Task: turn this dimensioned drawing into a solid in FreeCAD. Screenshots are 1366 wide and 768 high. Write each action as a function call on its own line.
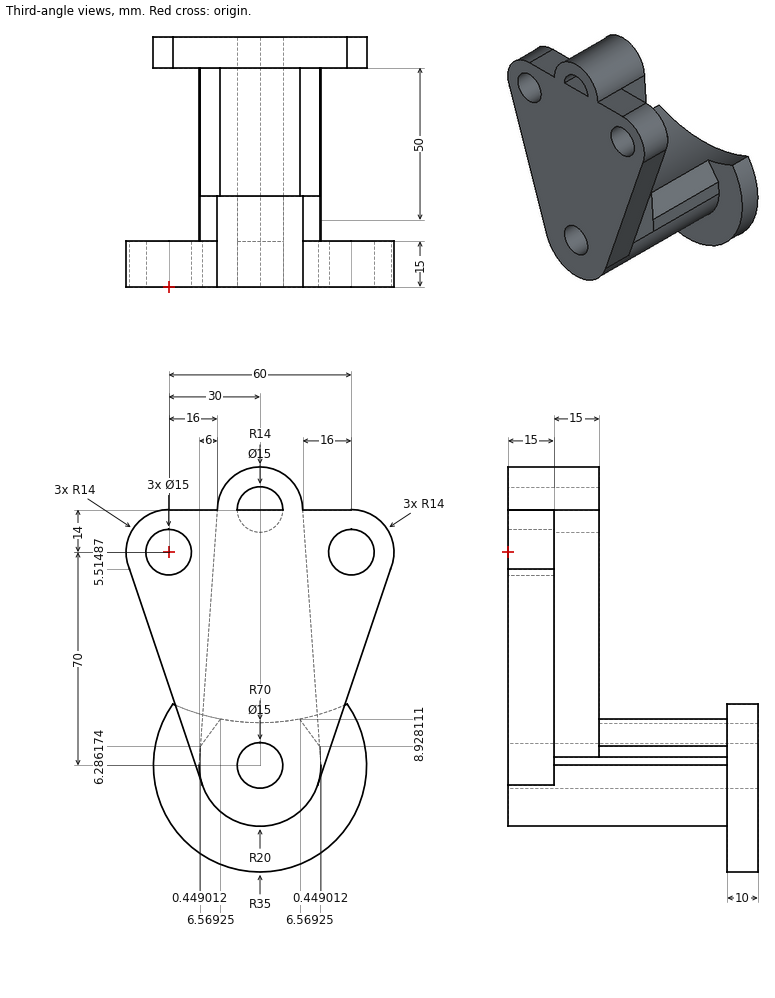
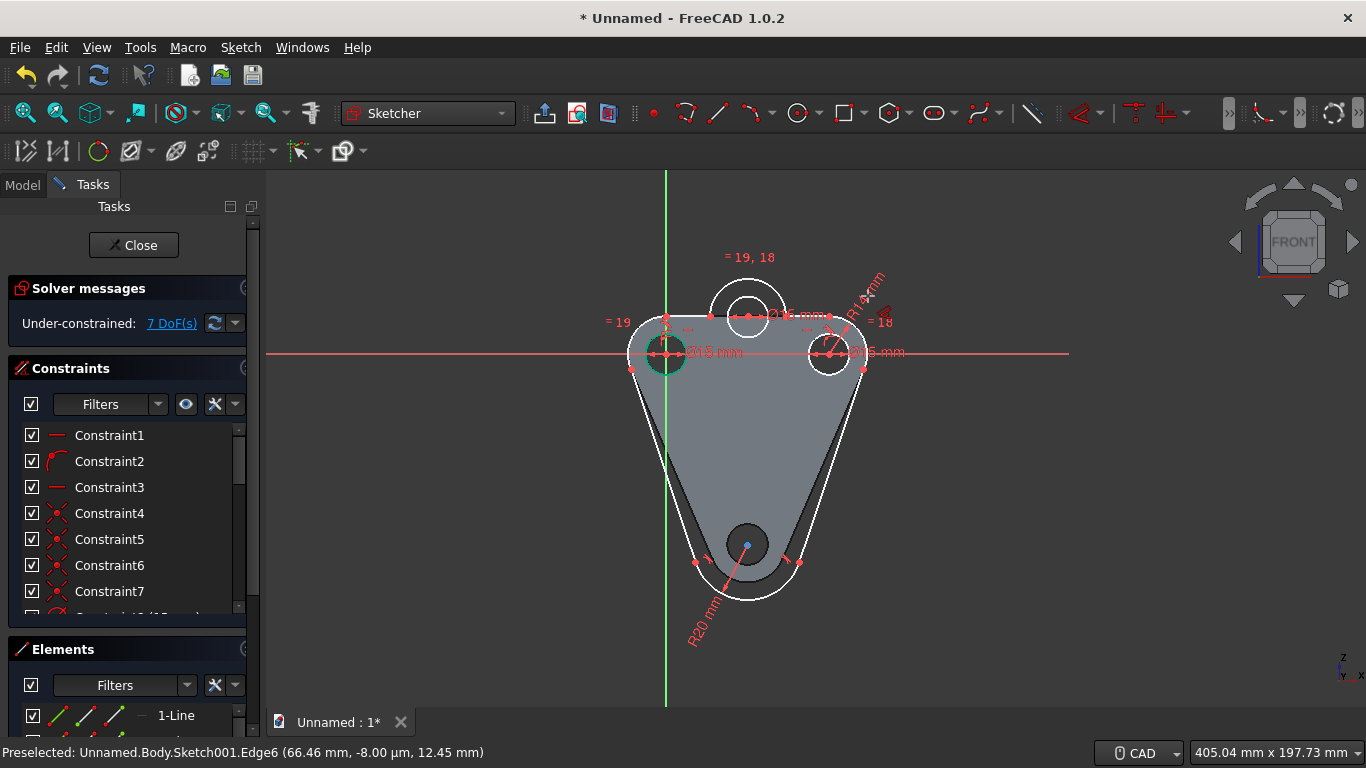
click(816, 316)
click(798, 282)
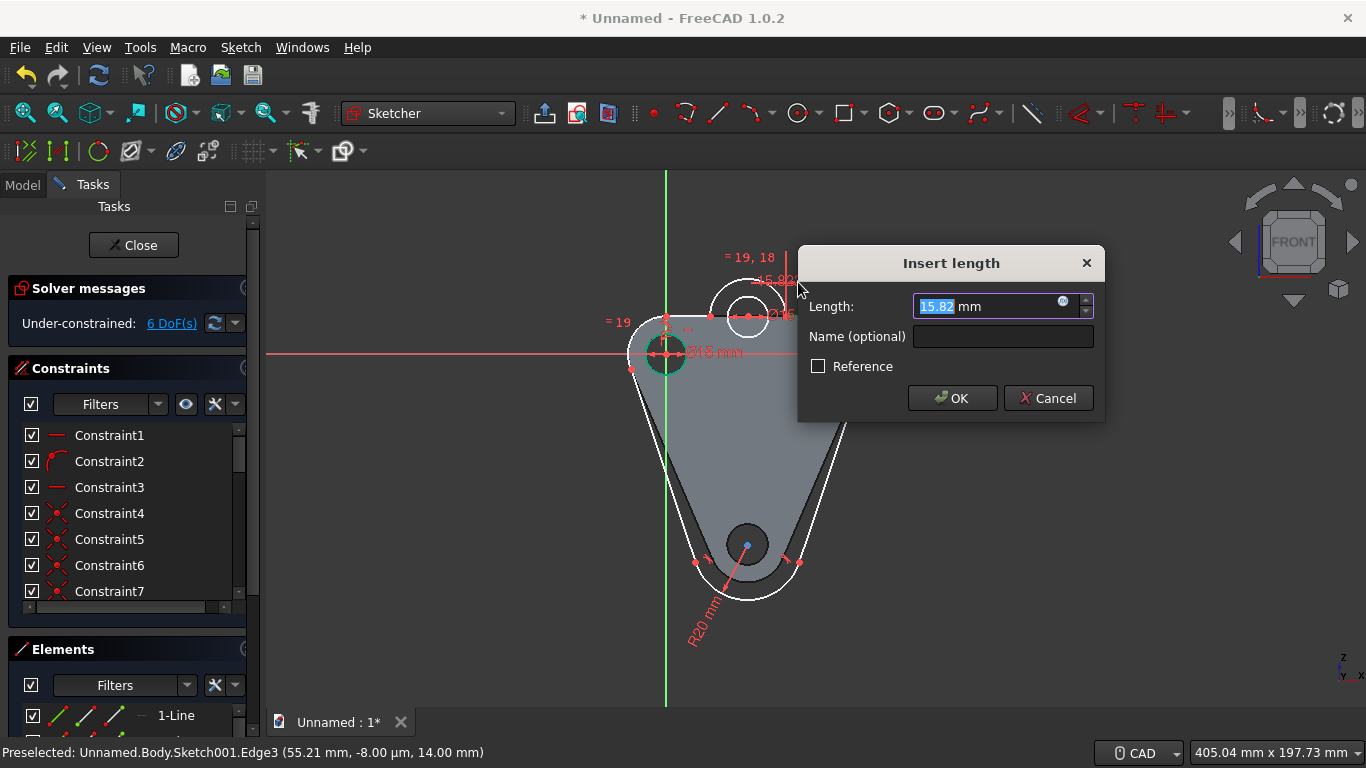
text(16)
key(Return)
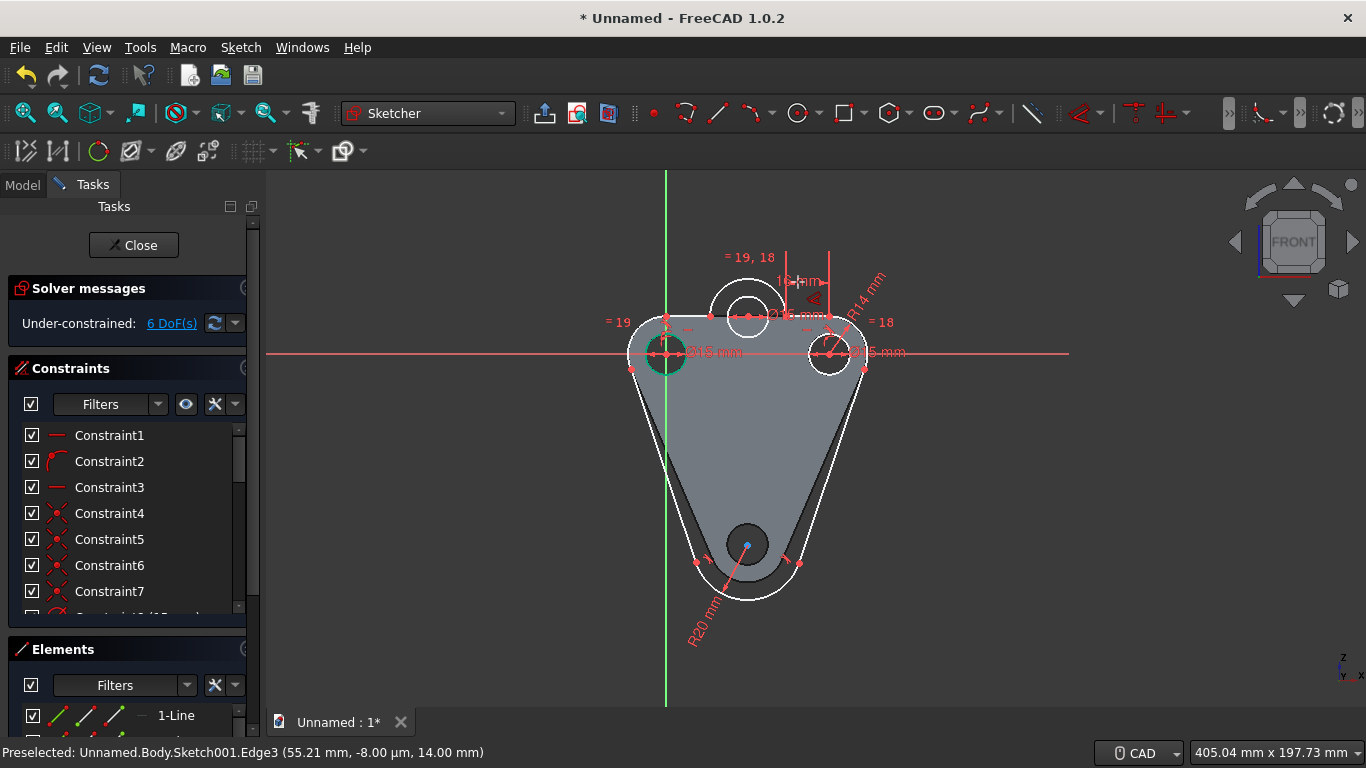
click(697, 316)
click(688, 282)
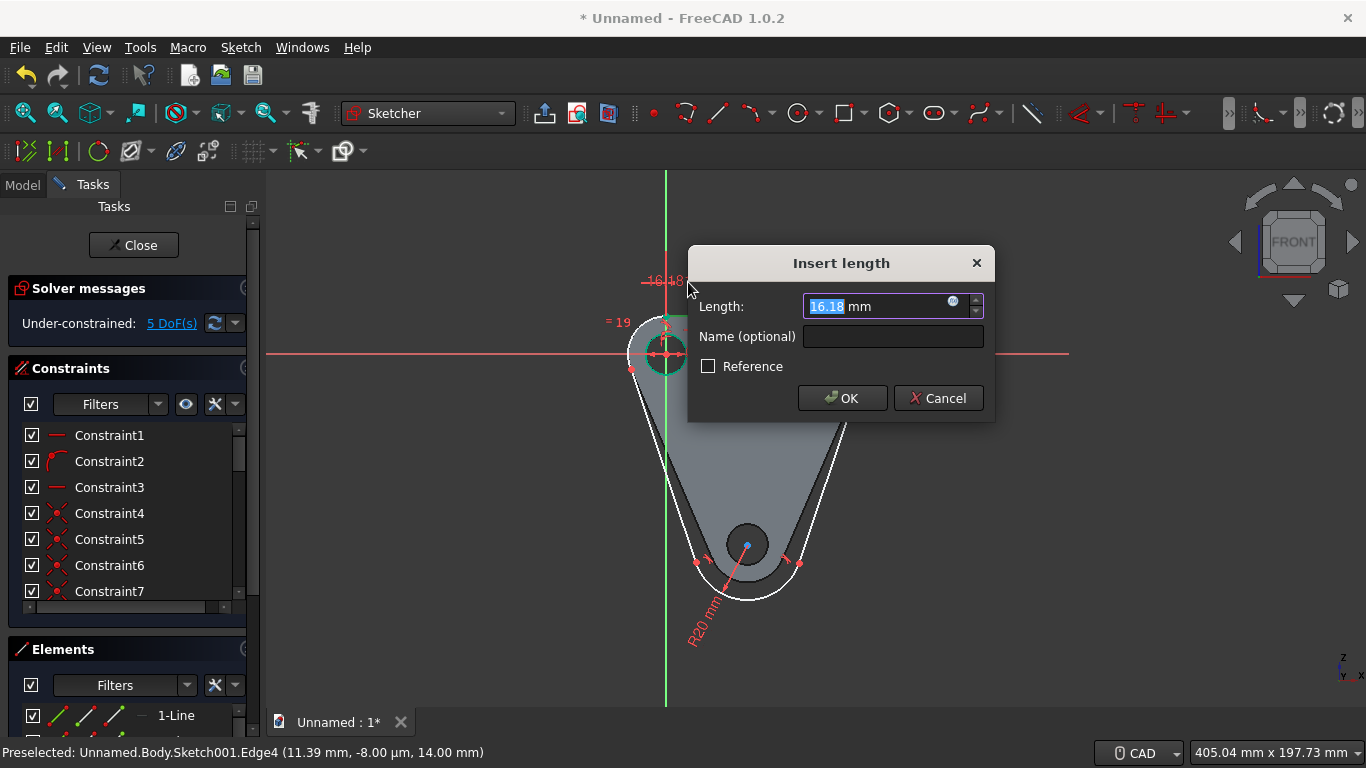
text(16)
key(Return)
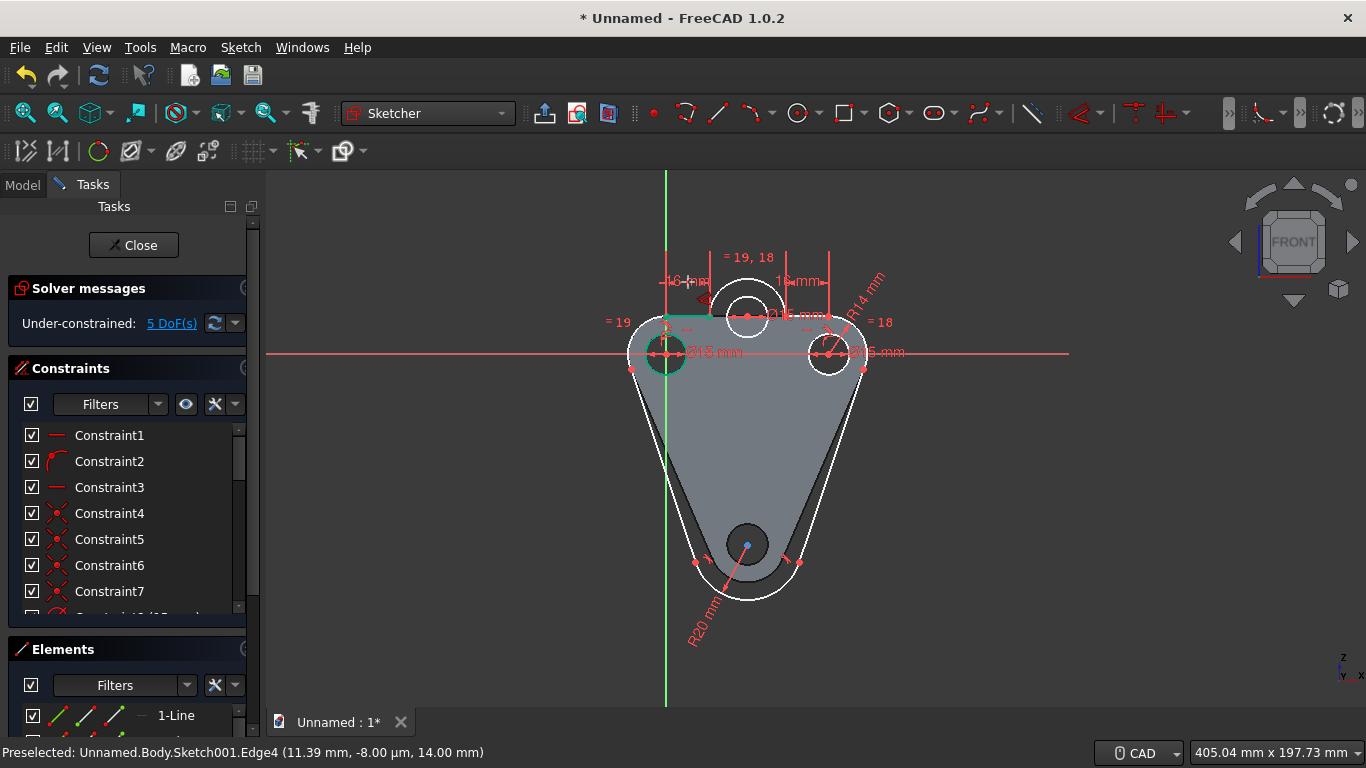
click(748, 317)
click(782, 336)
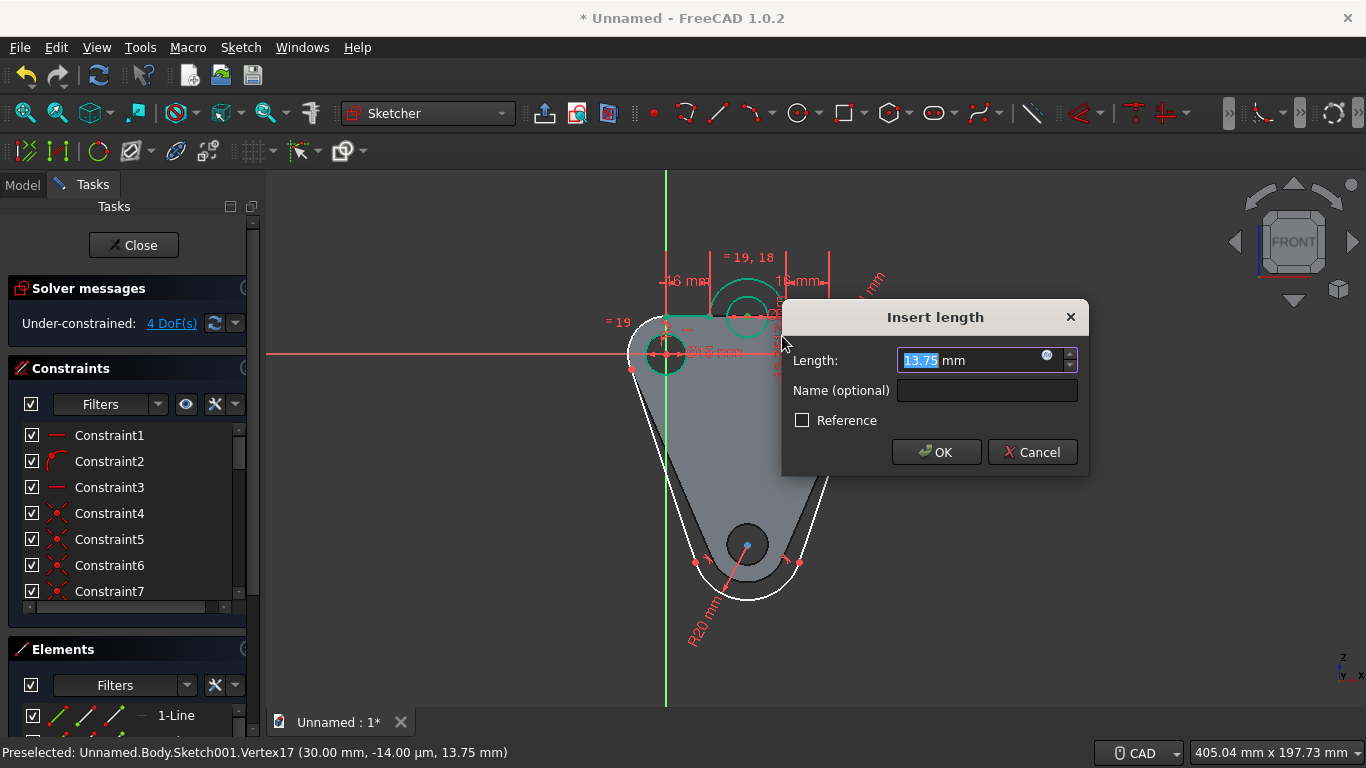
text(14)
key(Return)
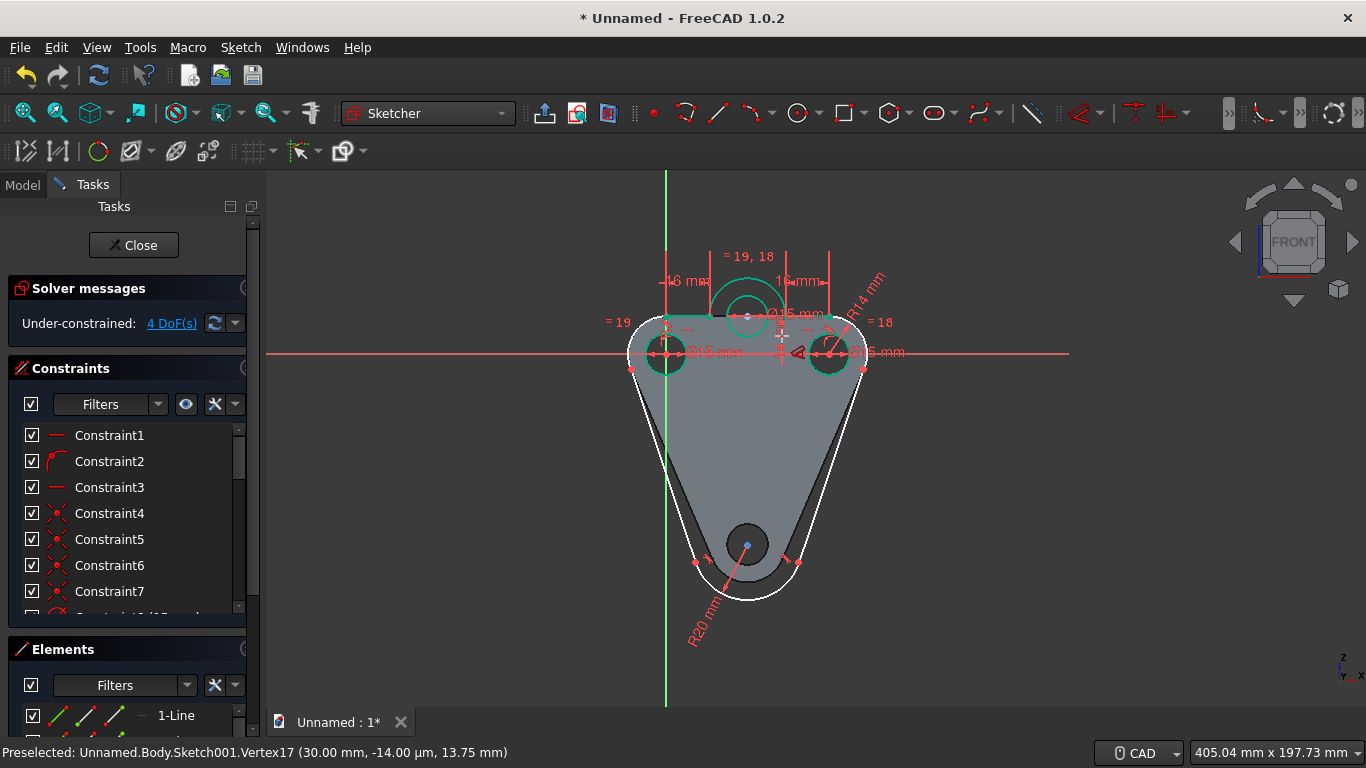
click(747, 546)
click(688, 580)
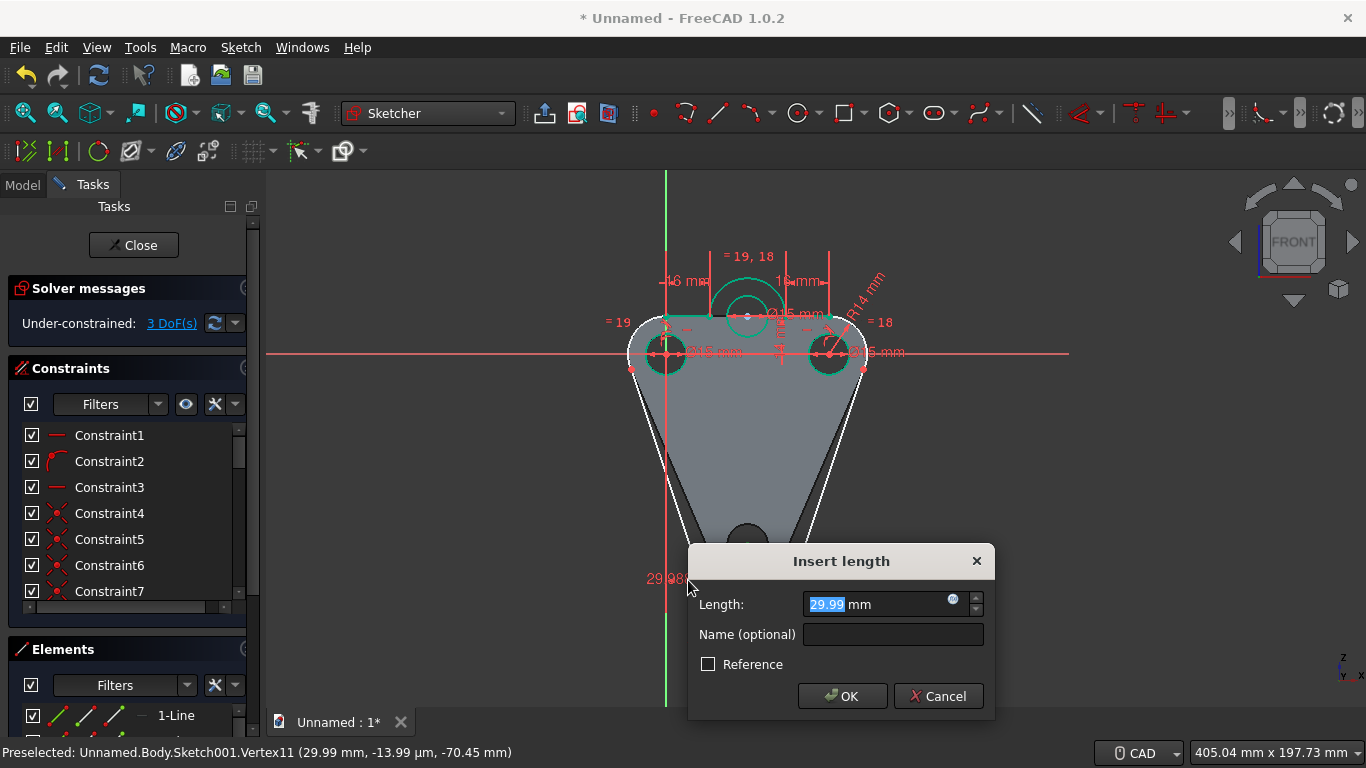
text(30)
key(Return)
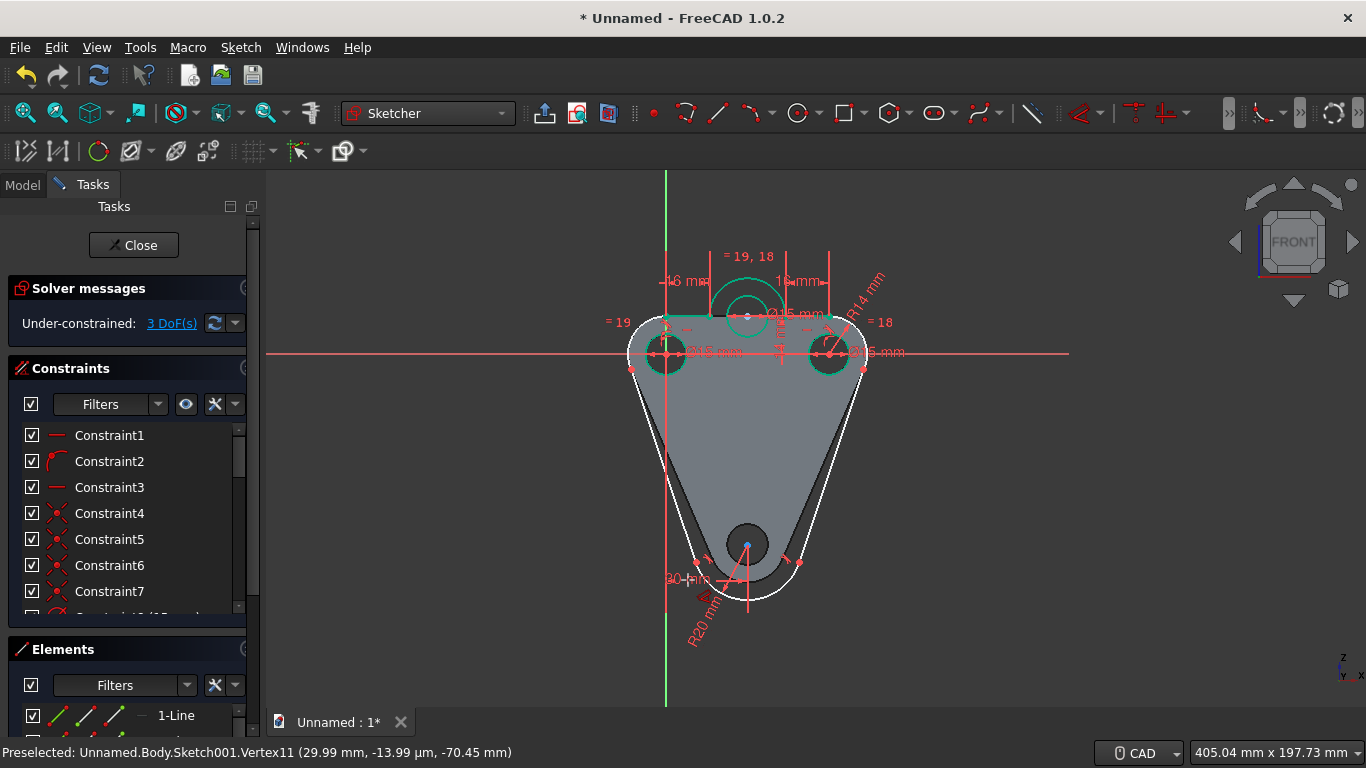
click(748, 546)
click(632, 450)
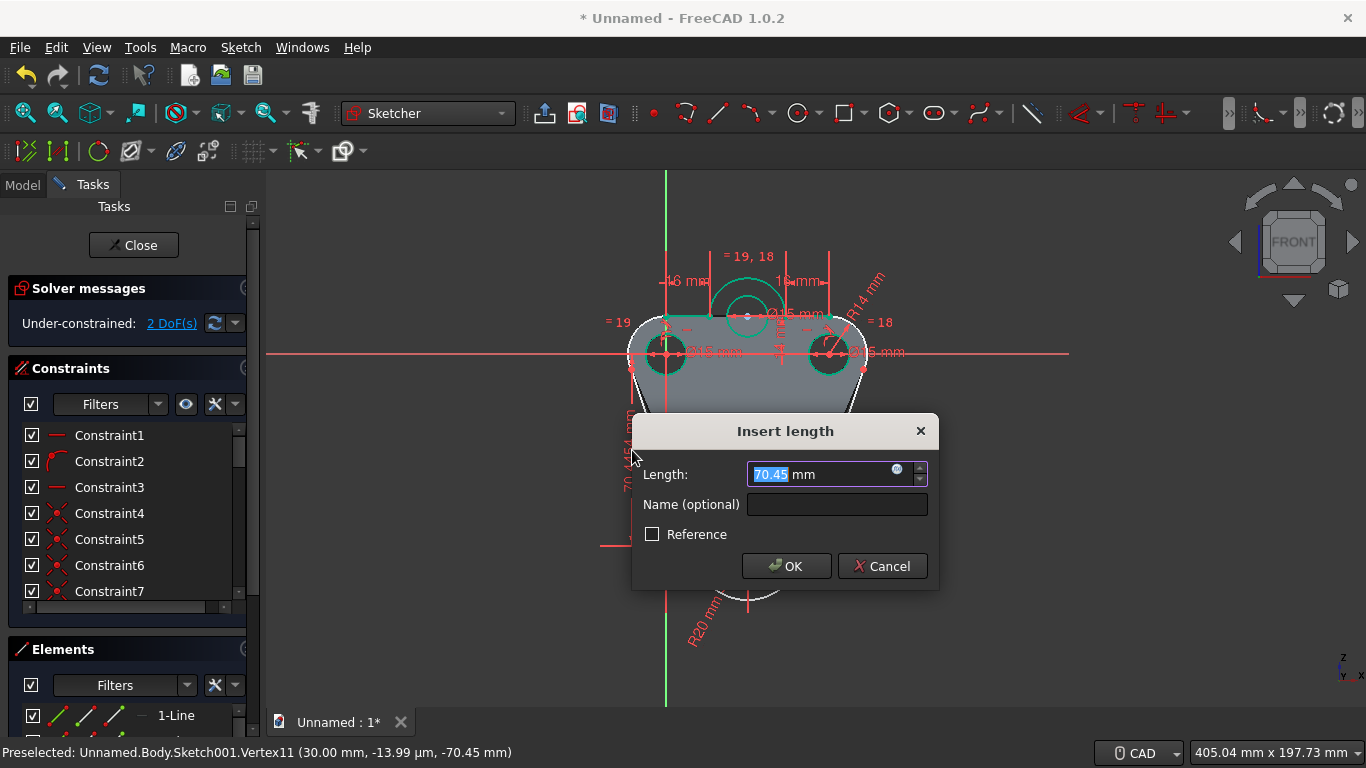
text(70)
key(Return)